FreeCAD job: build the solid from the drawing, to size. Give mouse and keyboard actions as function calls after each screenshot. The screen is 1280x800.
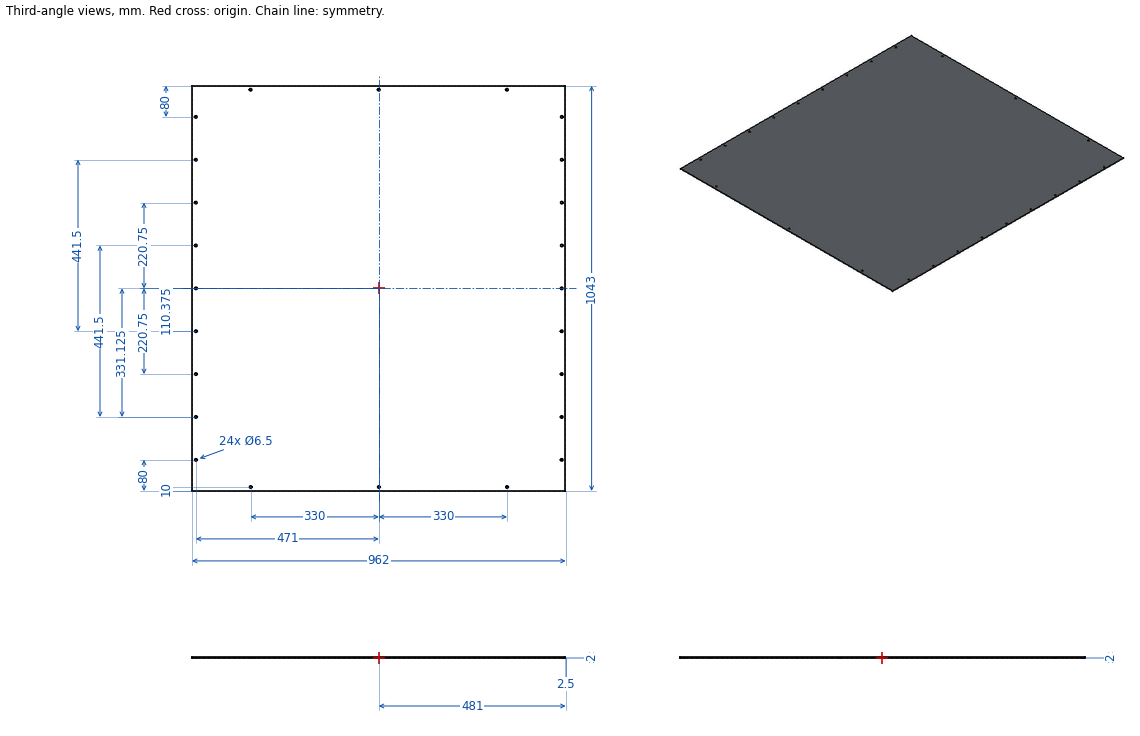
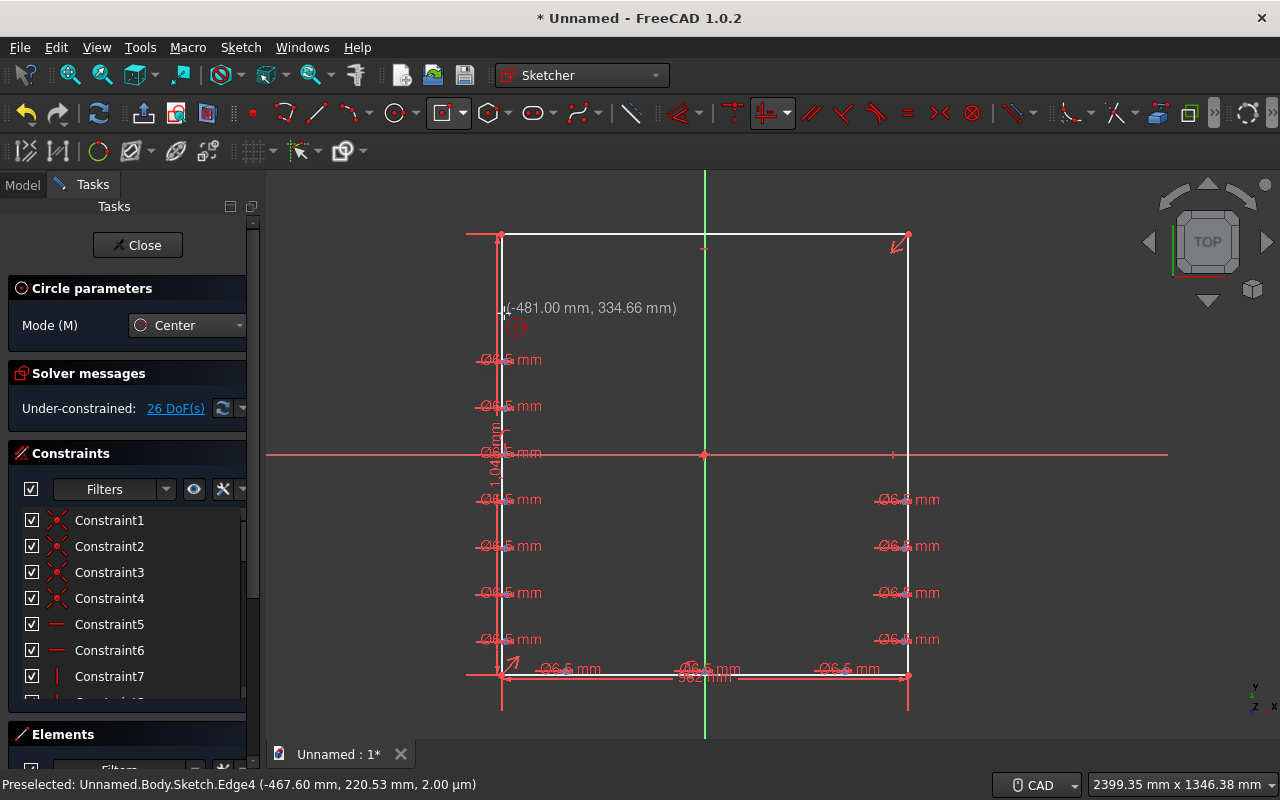
scroll(506, 315, up, 7)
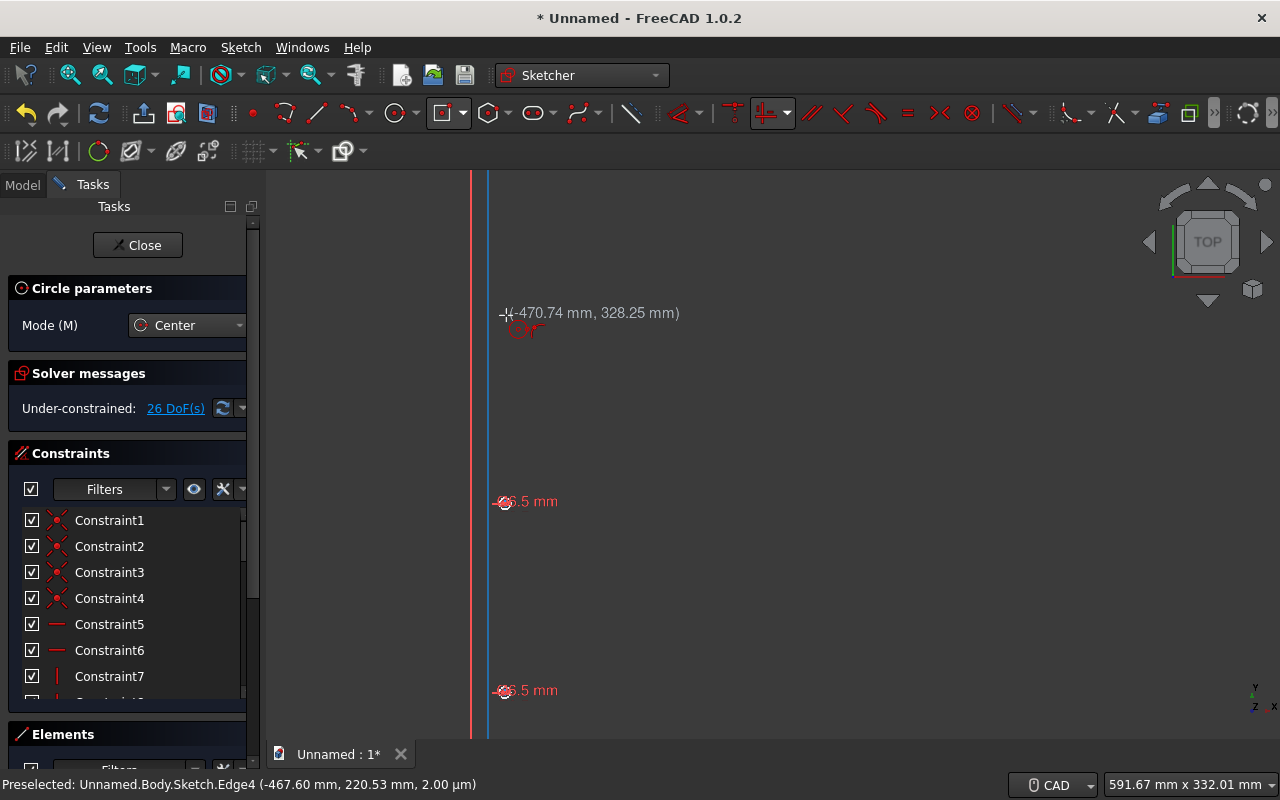
click(505, 313)
move(509, 309)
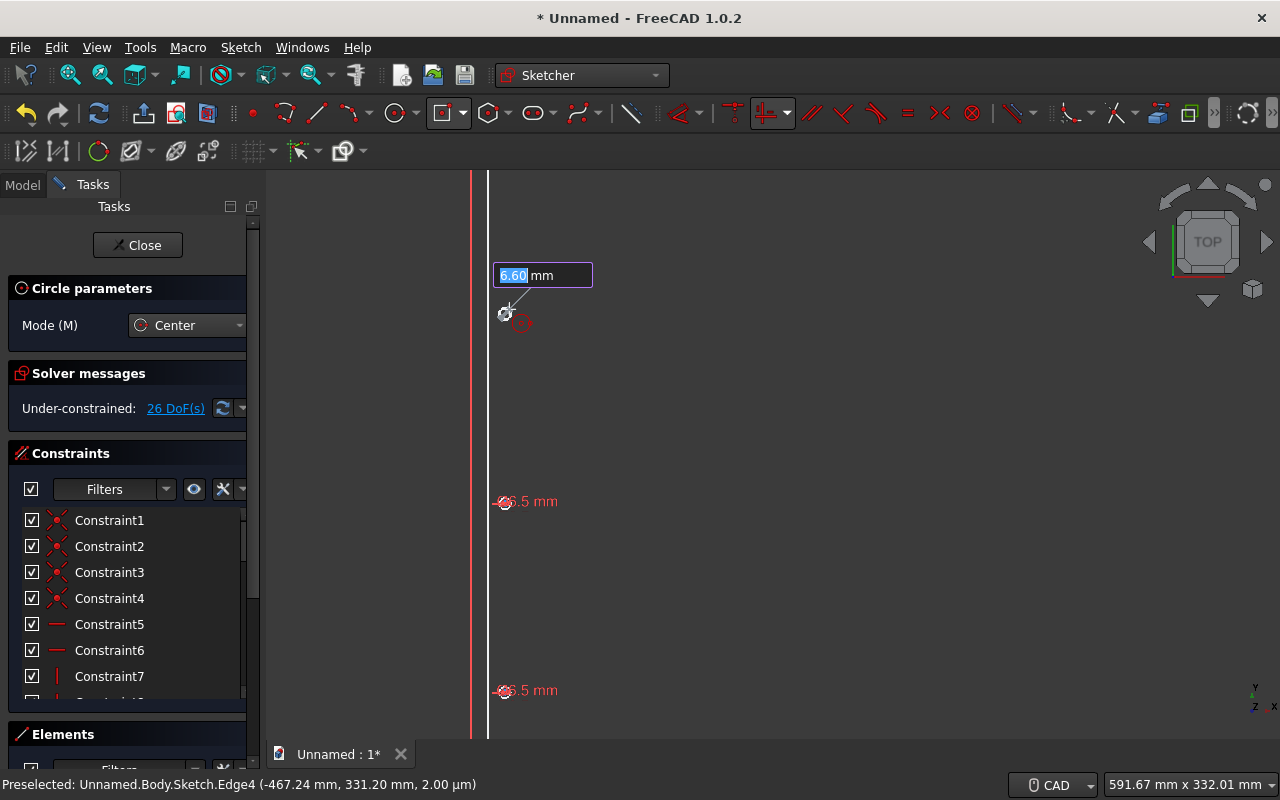
text(6.5)
key(Return)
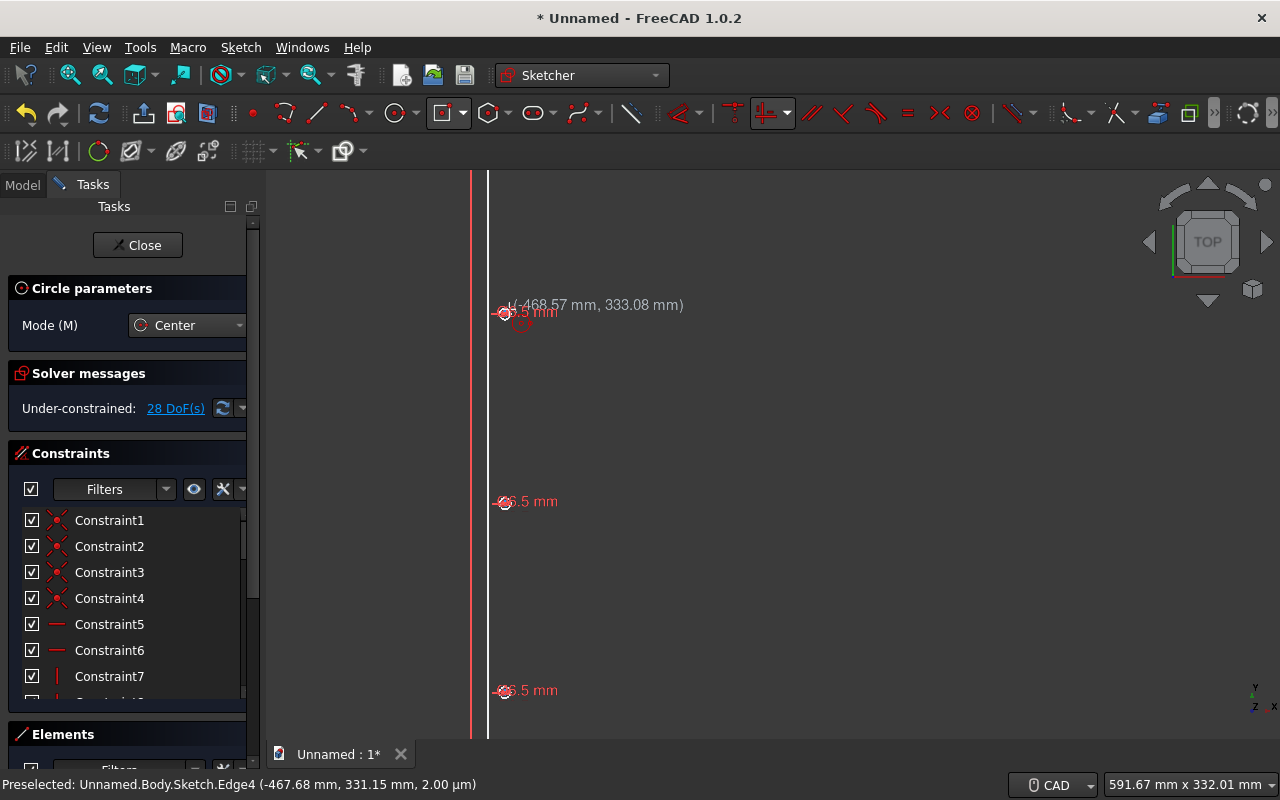
scroll(551, 347, down, 8)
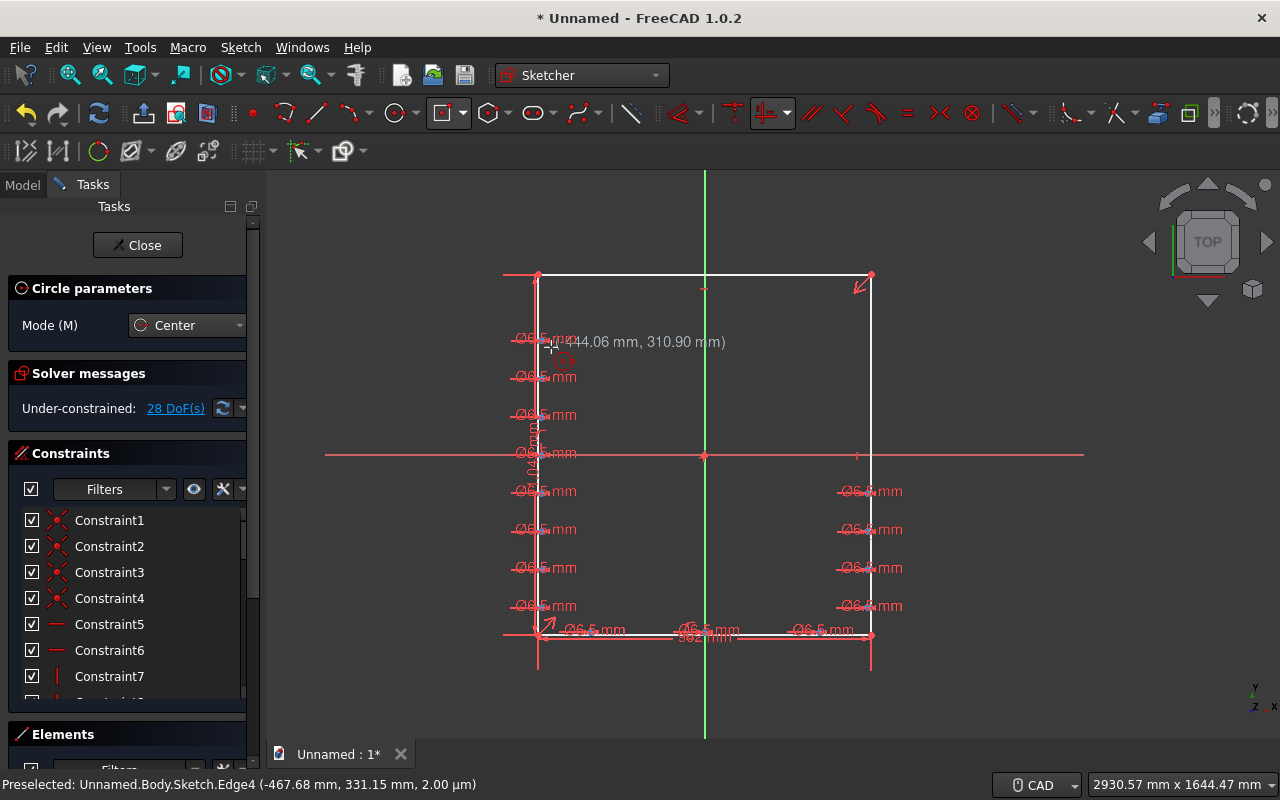
scroll(542, 302, up, 16)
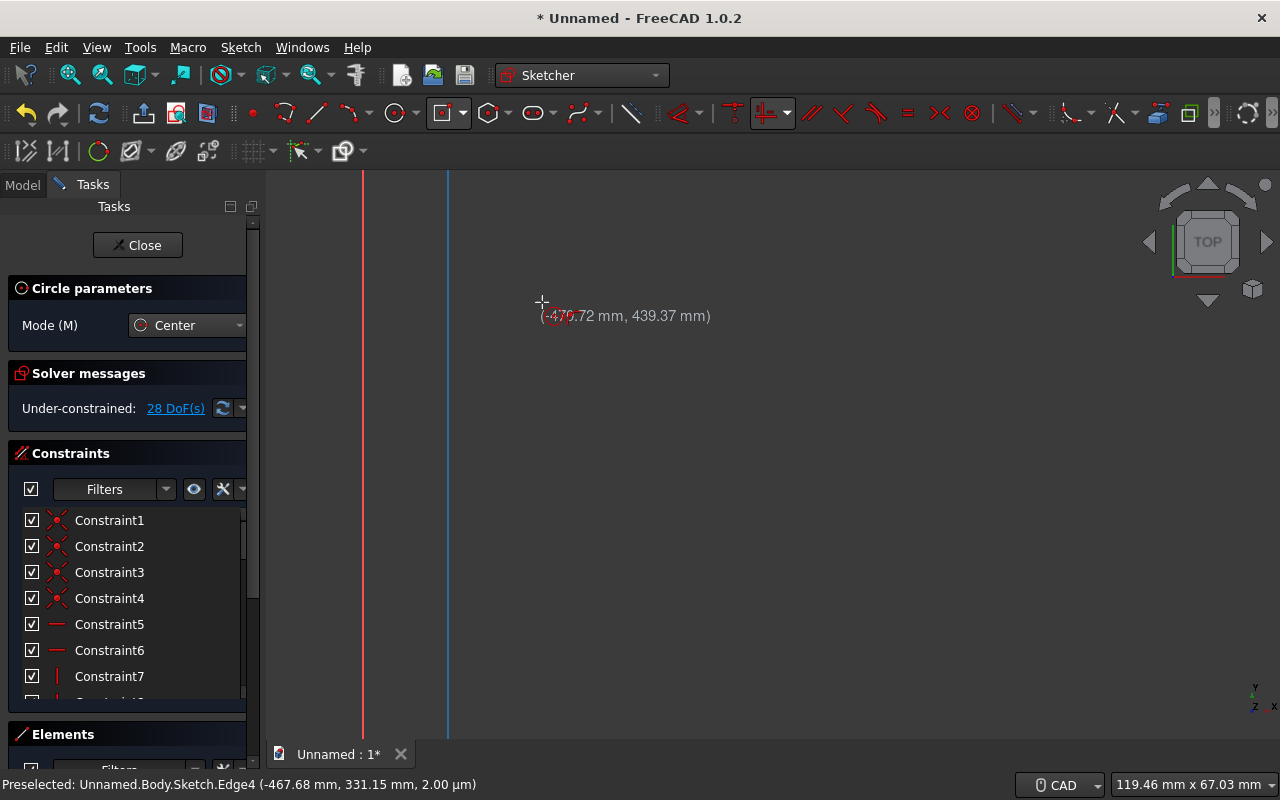
scroll(504, 266, down, 15)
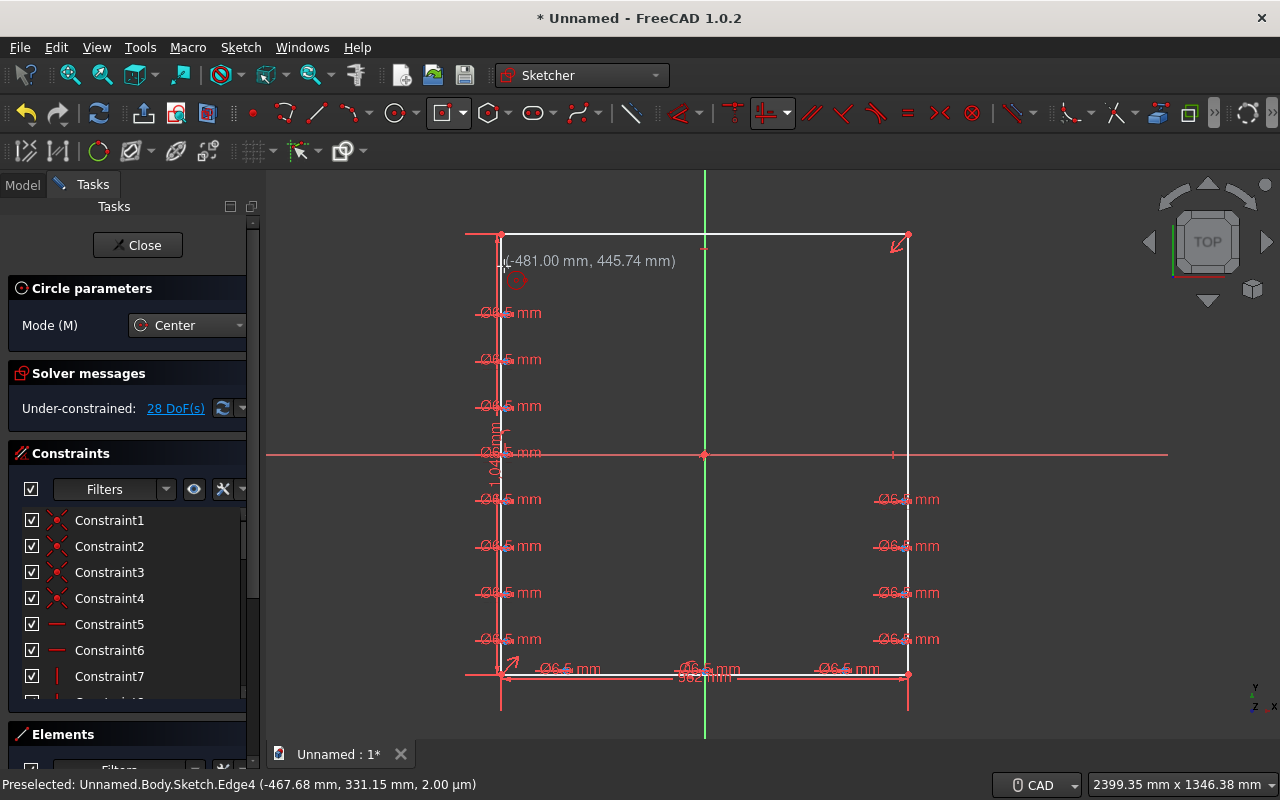
scroll(506, 268, up, 7)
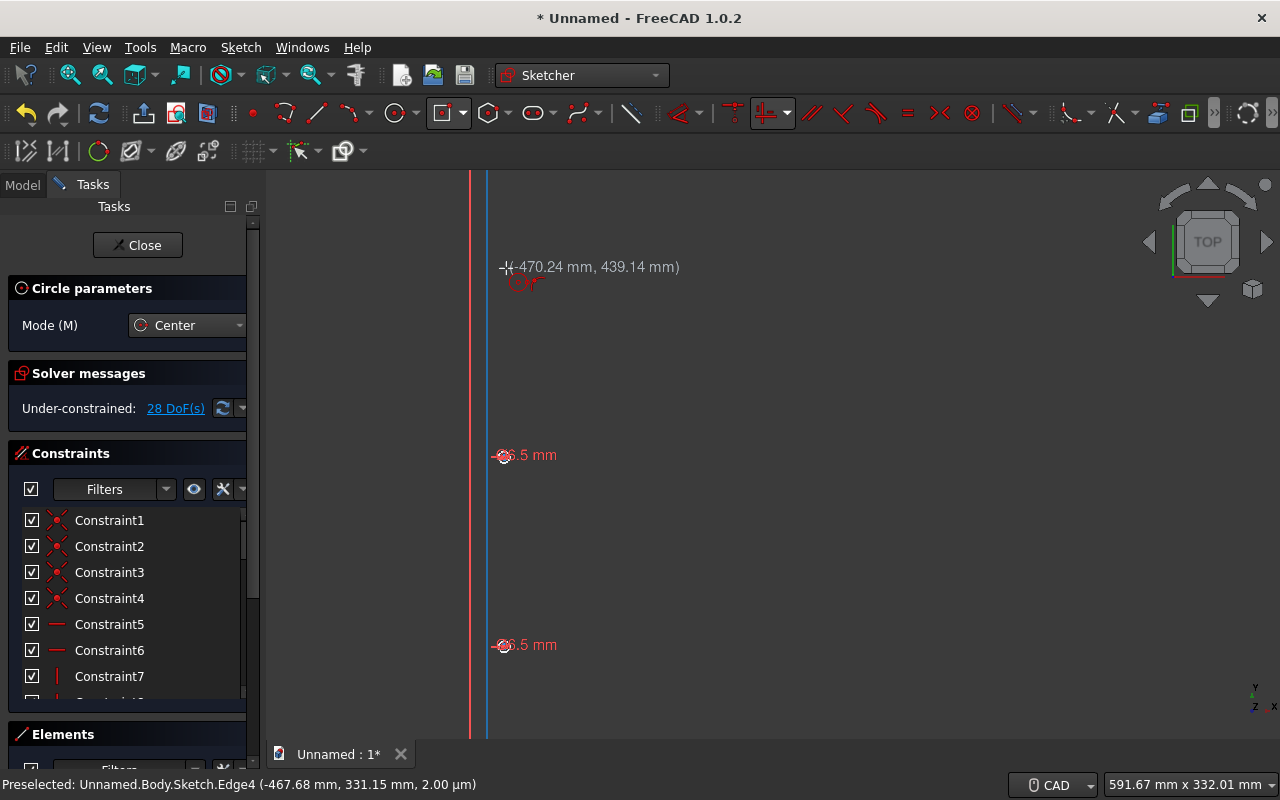
click(504, 267)
move(508, 264)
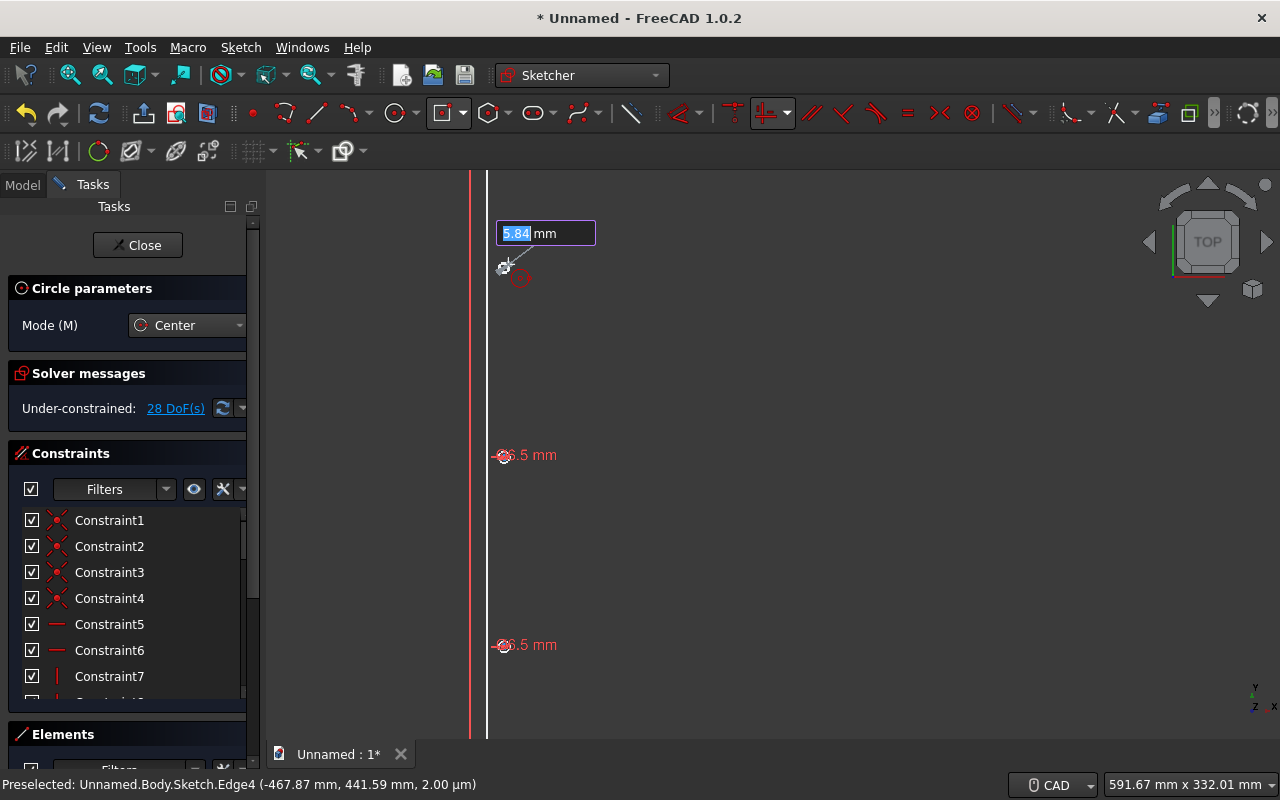
text(6.5)
key(Return)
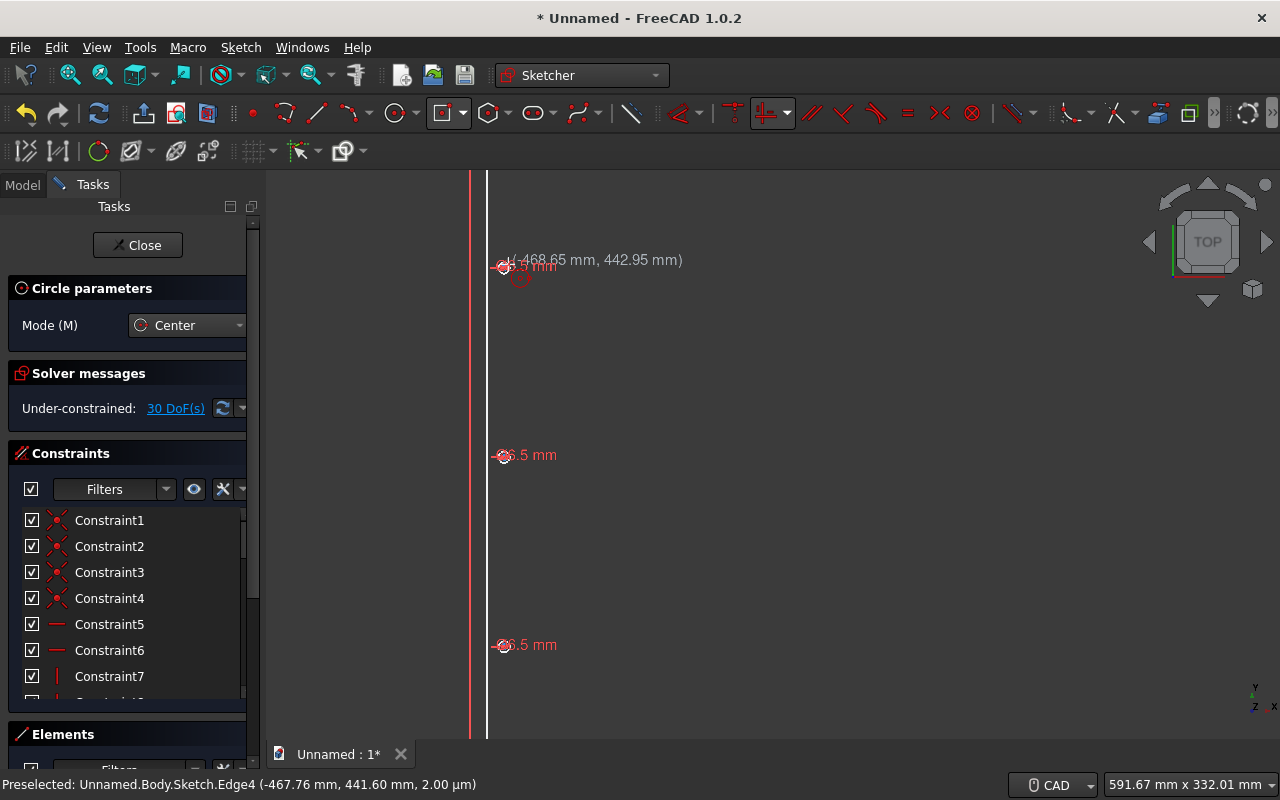
scroll(551, 310, down, 8)